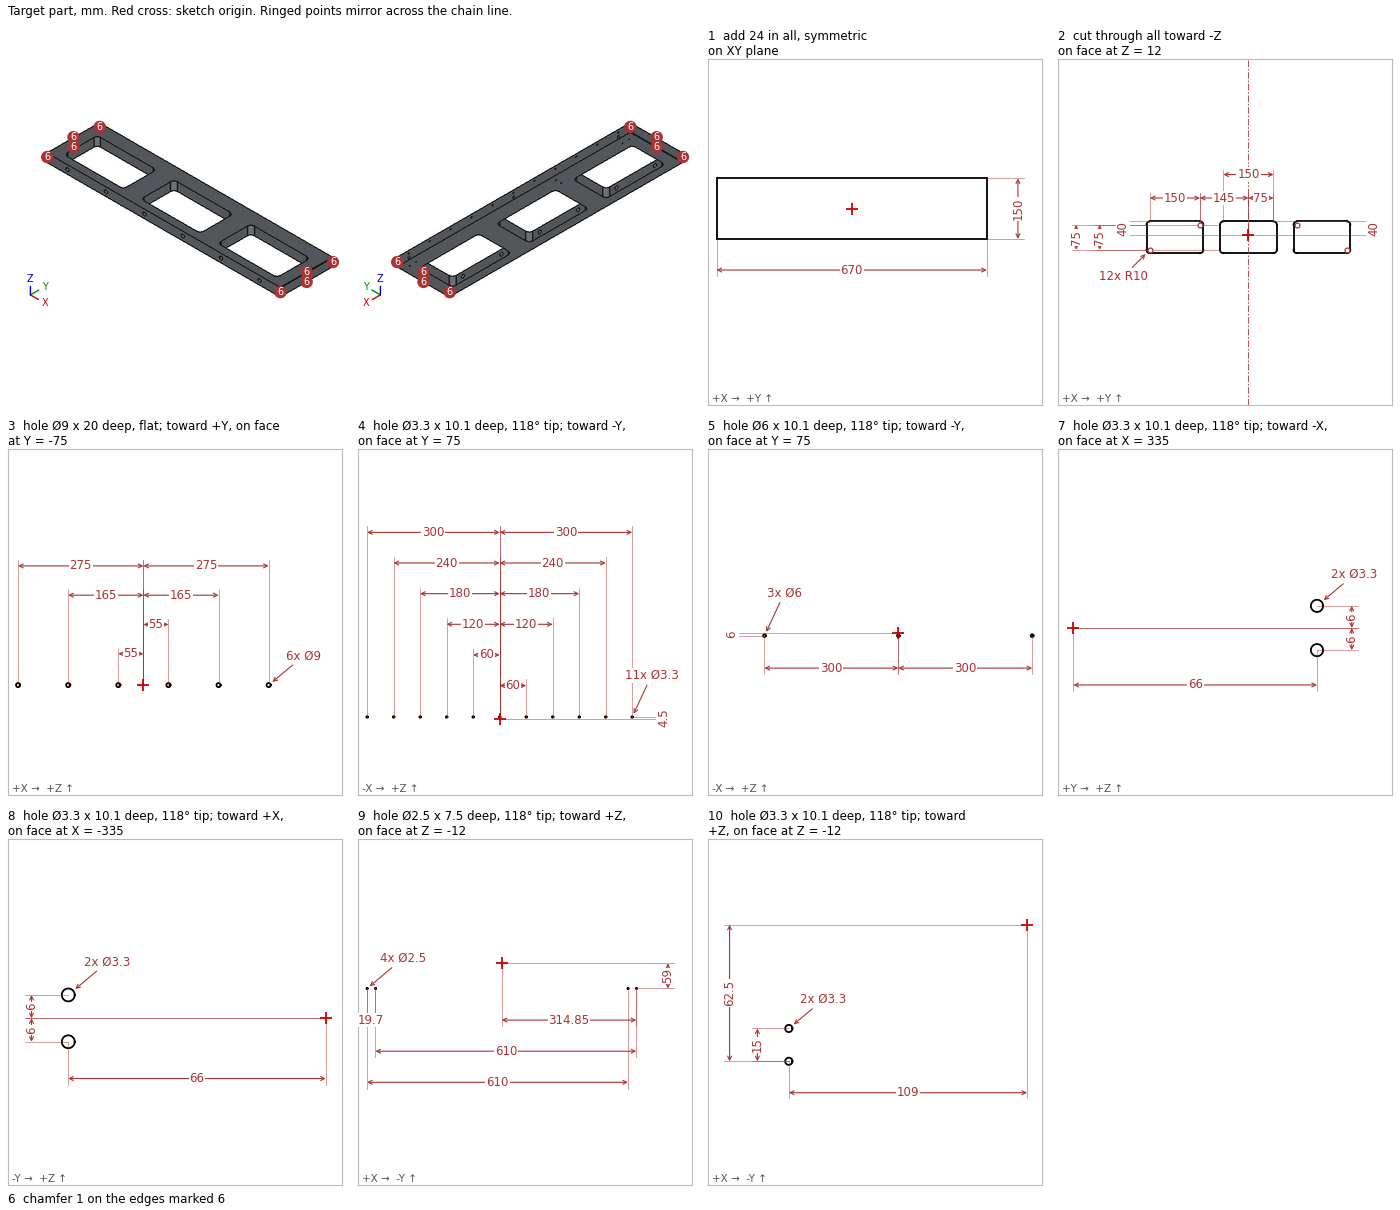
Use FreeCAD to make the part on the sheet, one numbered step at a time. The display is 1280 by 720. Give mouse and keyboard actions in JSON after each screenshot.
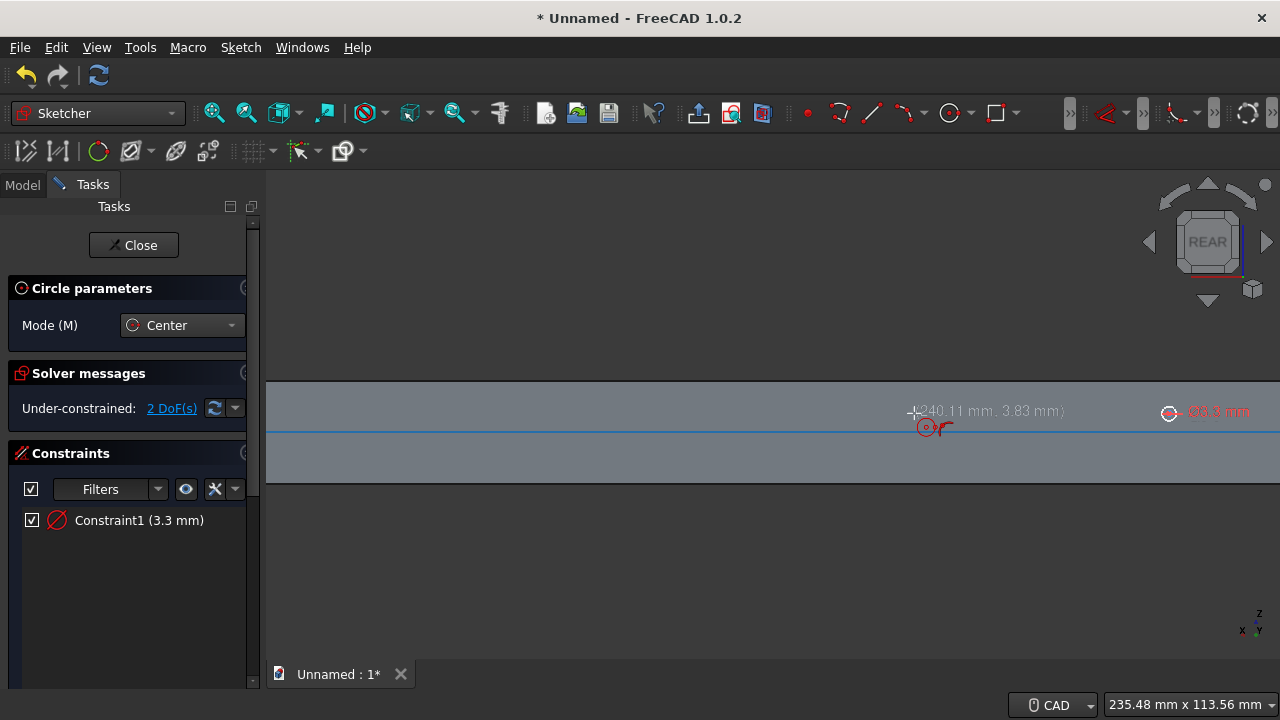
{"action": "left_click", "coordinate": [911, 413]}
{"action": "mouse_move", "coordinate": [916, 408]}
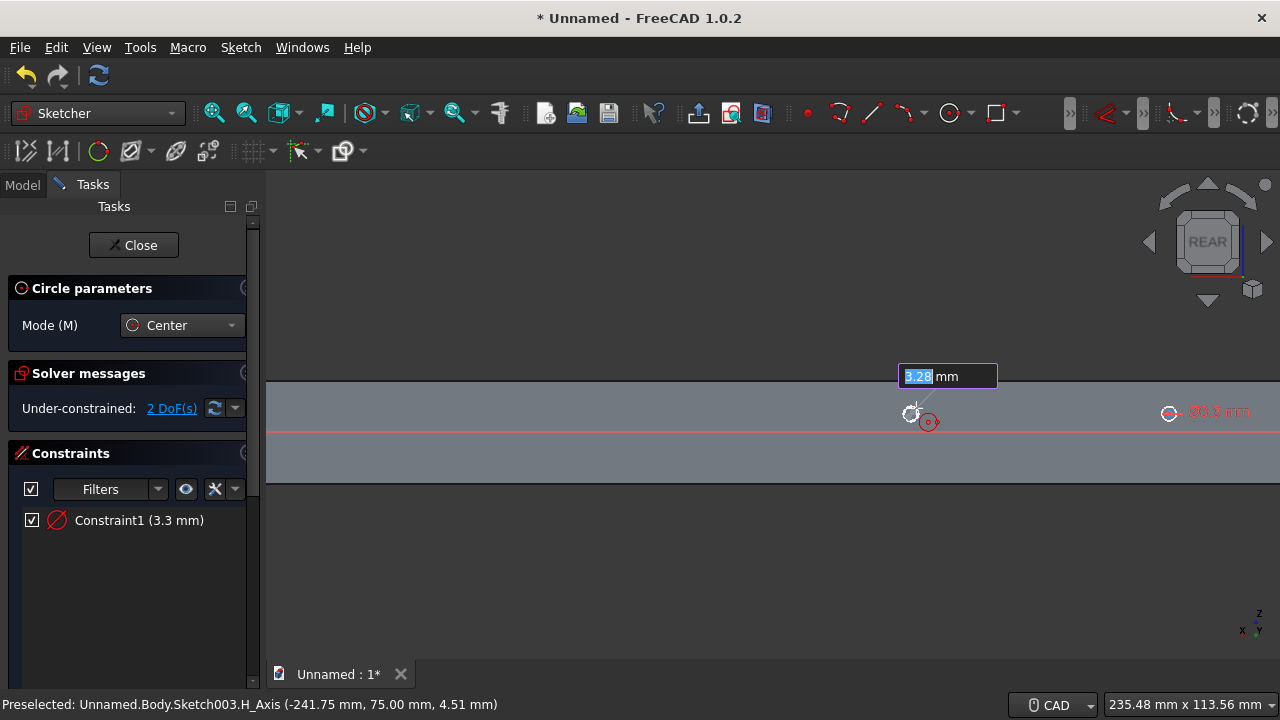
{"action": "type", "text": "3.3"}
{"action": "key", "text": "Return"}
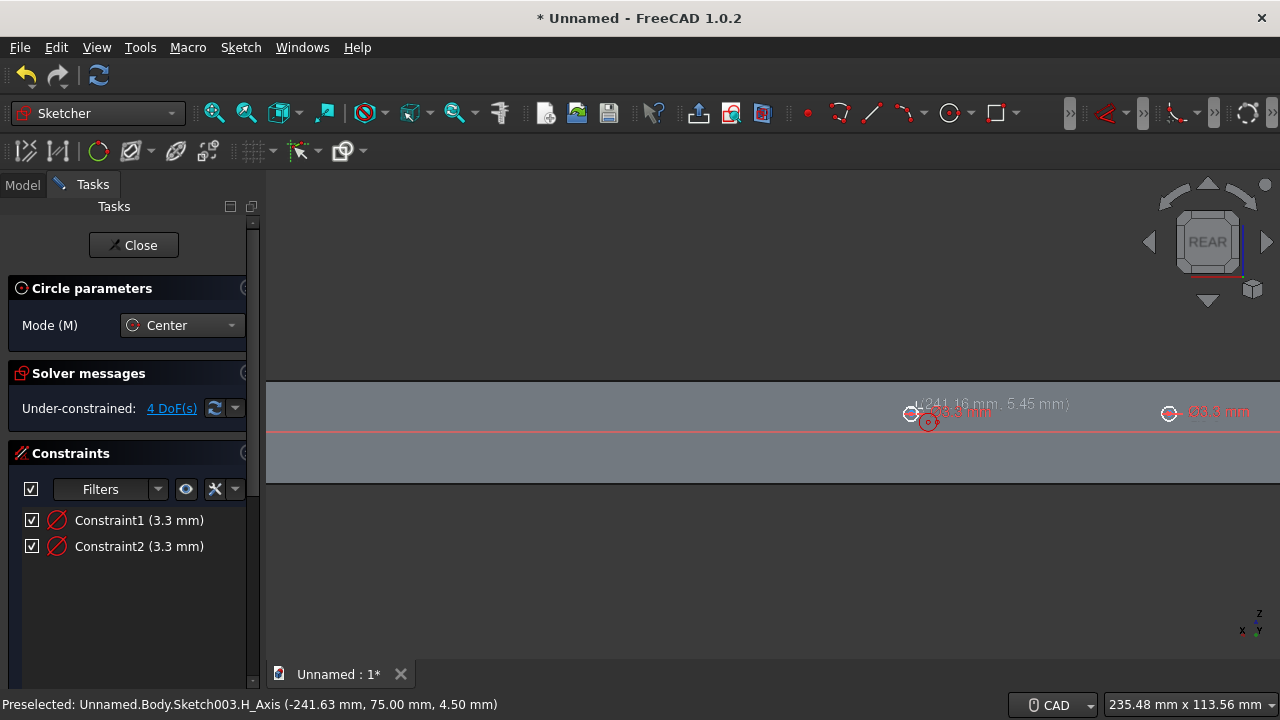
{"action": "scroll", "coordinate": [653, 413], "scroll_direction": "up", "scroll_amount": 6}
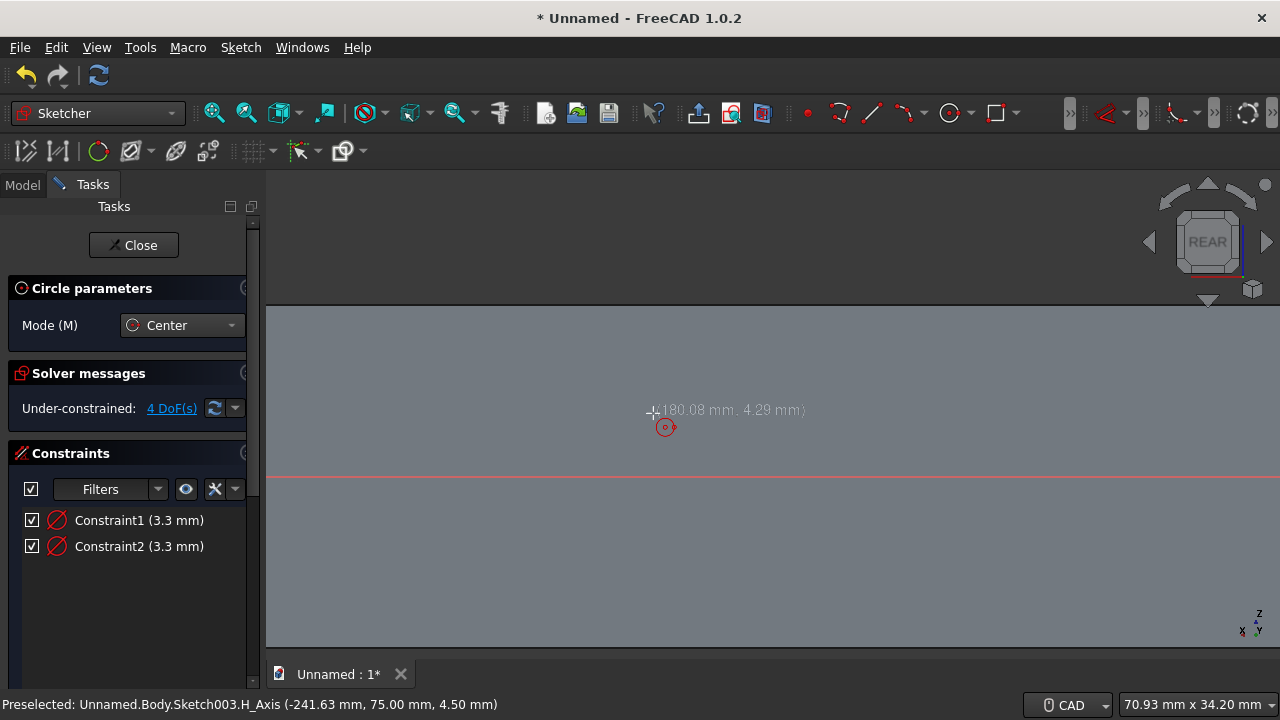
{"action": "scroll", "coordinate": [875, 413], "scroll_direction": "down", "scroll_amount": 14}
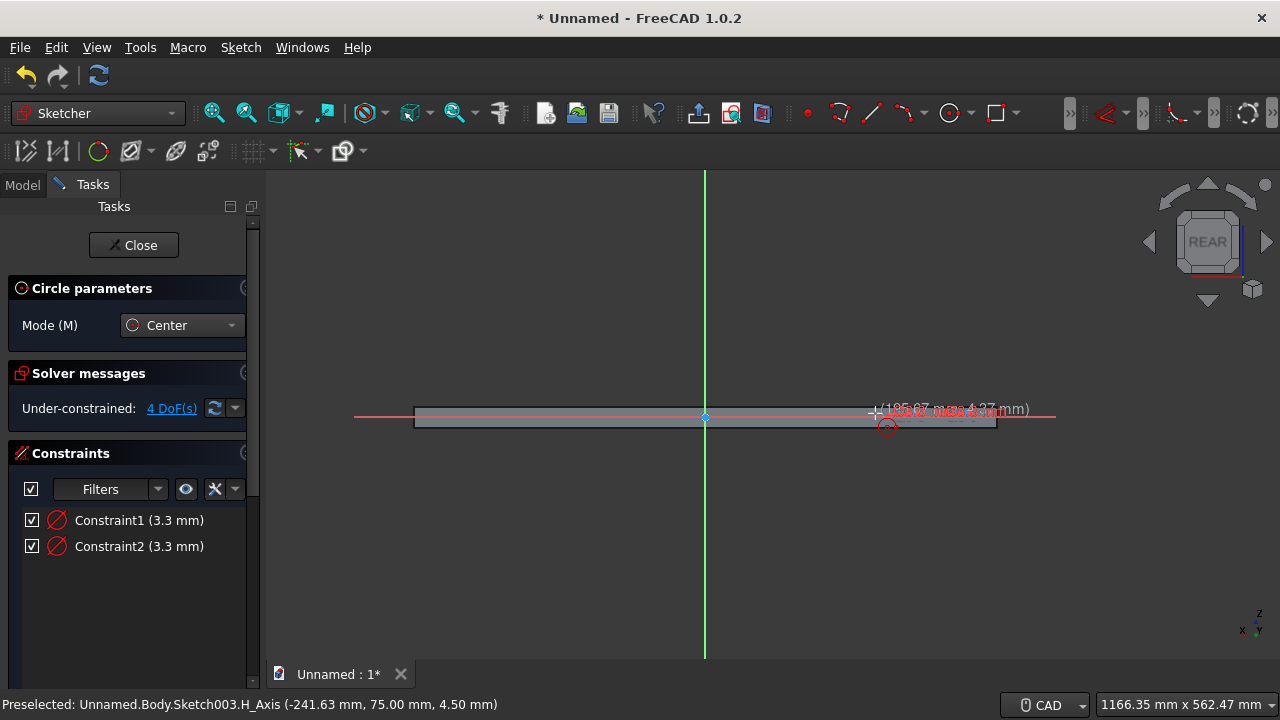
{"action": "scroll", "coordinate": [862, 413], "scroll_direction": "up", "scroll_amount": 8}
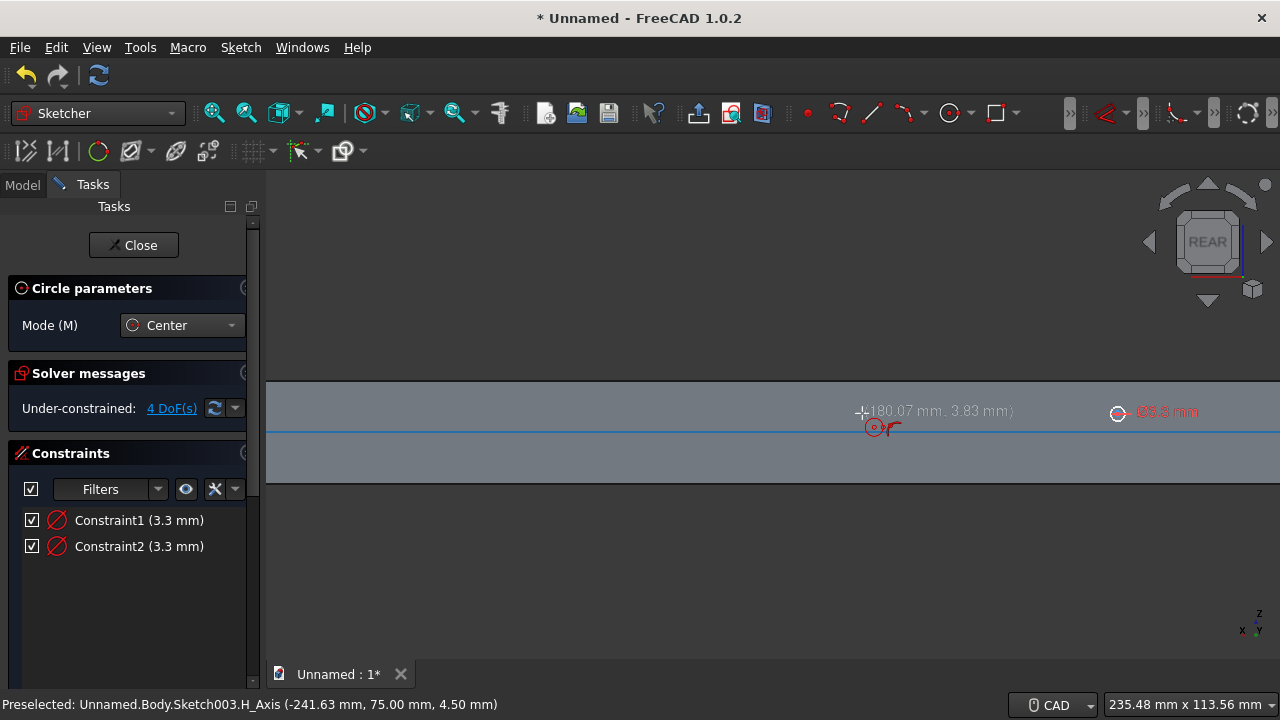
{"action": "left_click", "coordinate": [859, 413]}
{"action": "mouse_move", "coordinate": [864, 408]}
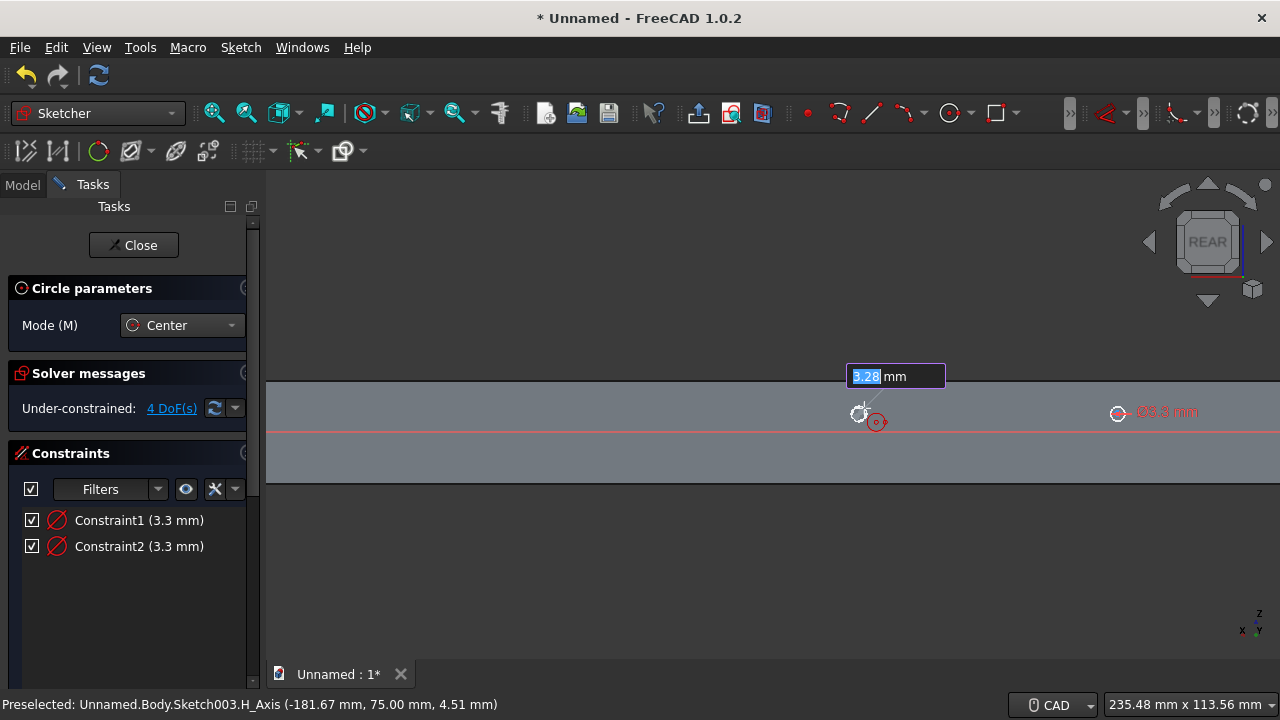
{"action": "type", "text": "3.3"}
{"action": "key", "text": "Return"}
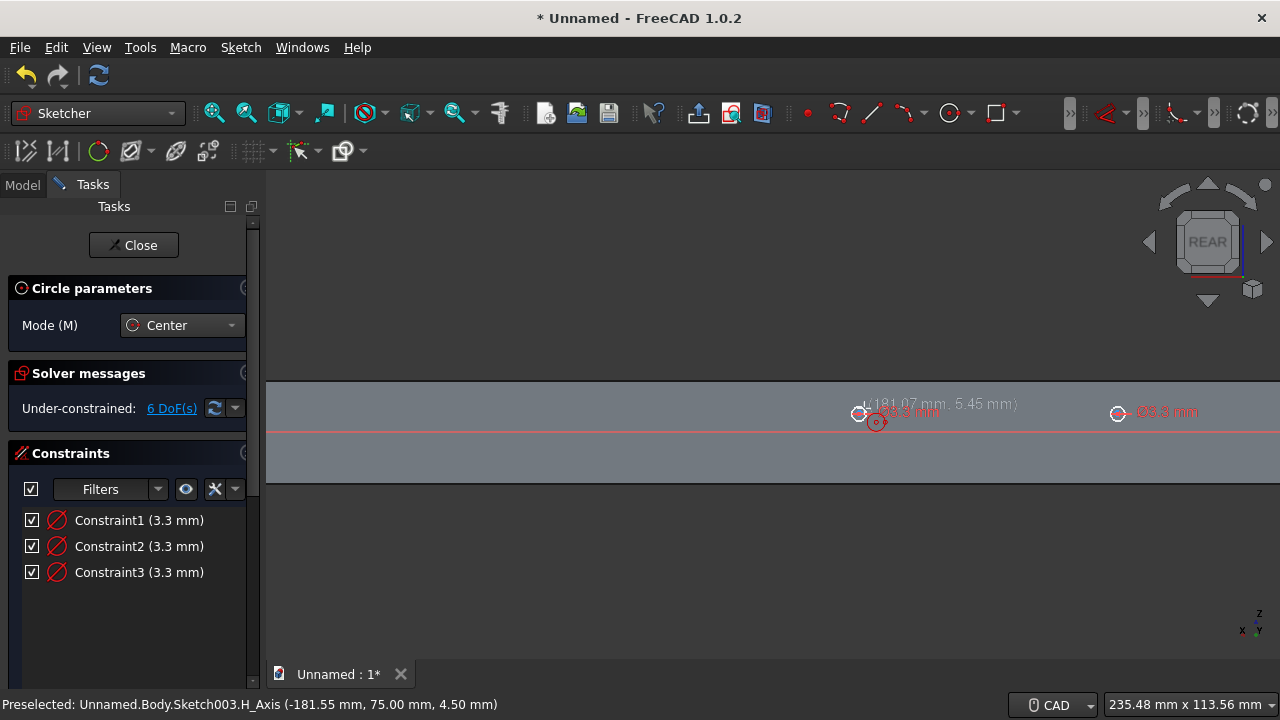
{"action": "scroll", "coordinate": [601, 413], "scroll_direction": "up", "scroll_amount": 6}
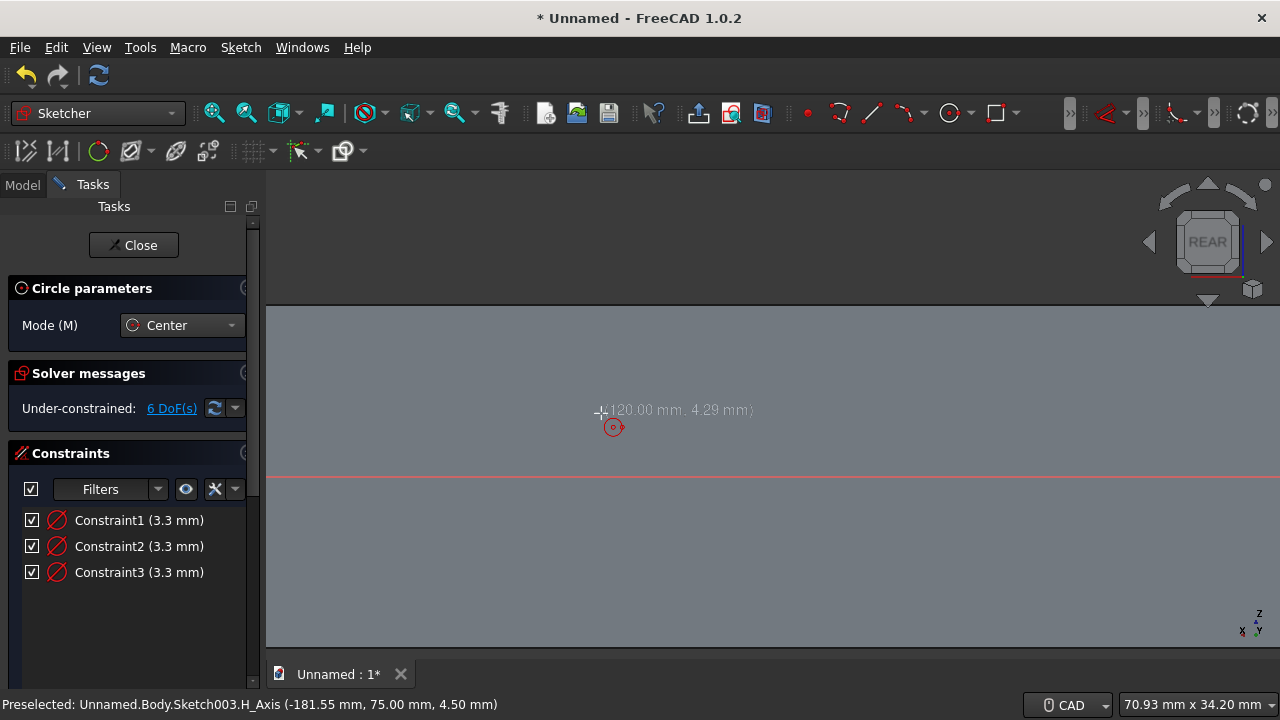
{"action": "scroll", "coordinate": [822, 413], "scroll_direction": "down", "scroll_amount": 14}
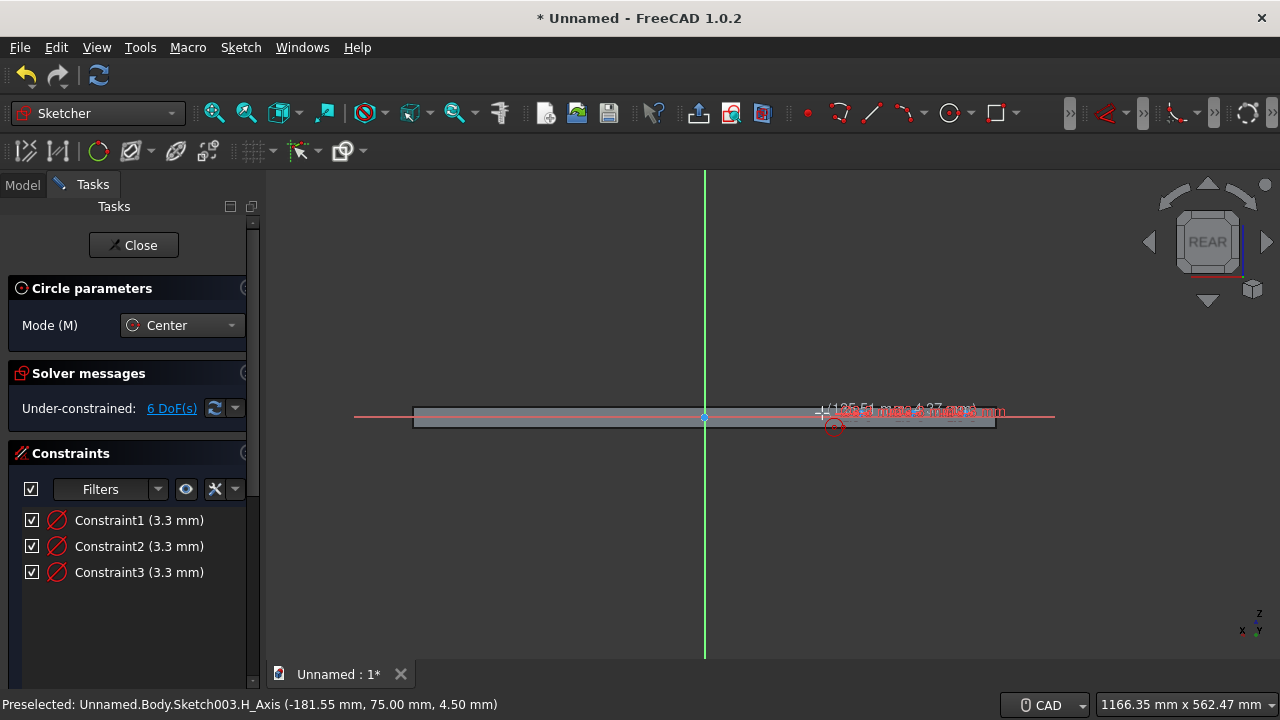
{"action": "scroll", "coordinate": [809, 413], "scroll_direction": "up", "scroll_amount": 8}